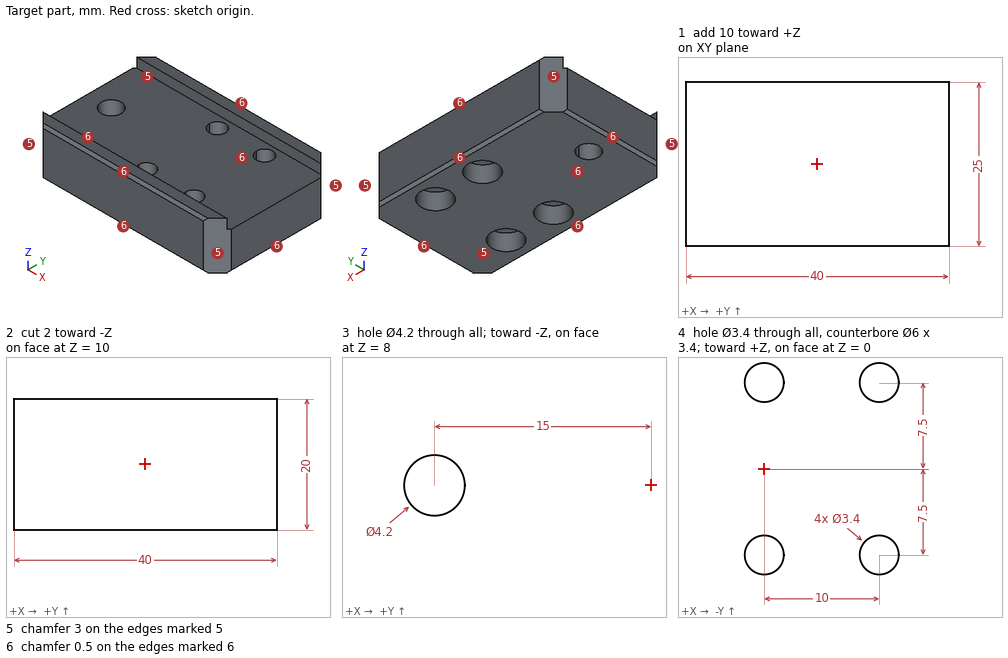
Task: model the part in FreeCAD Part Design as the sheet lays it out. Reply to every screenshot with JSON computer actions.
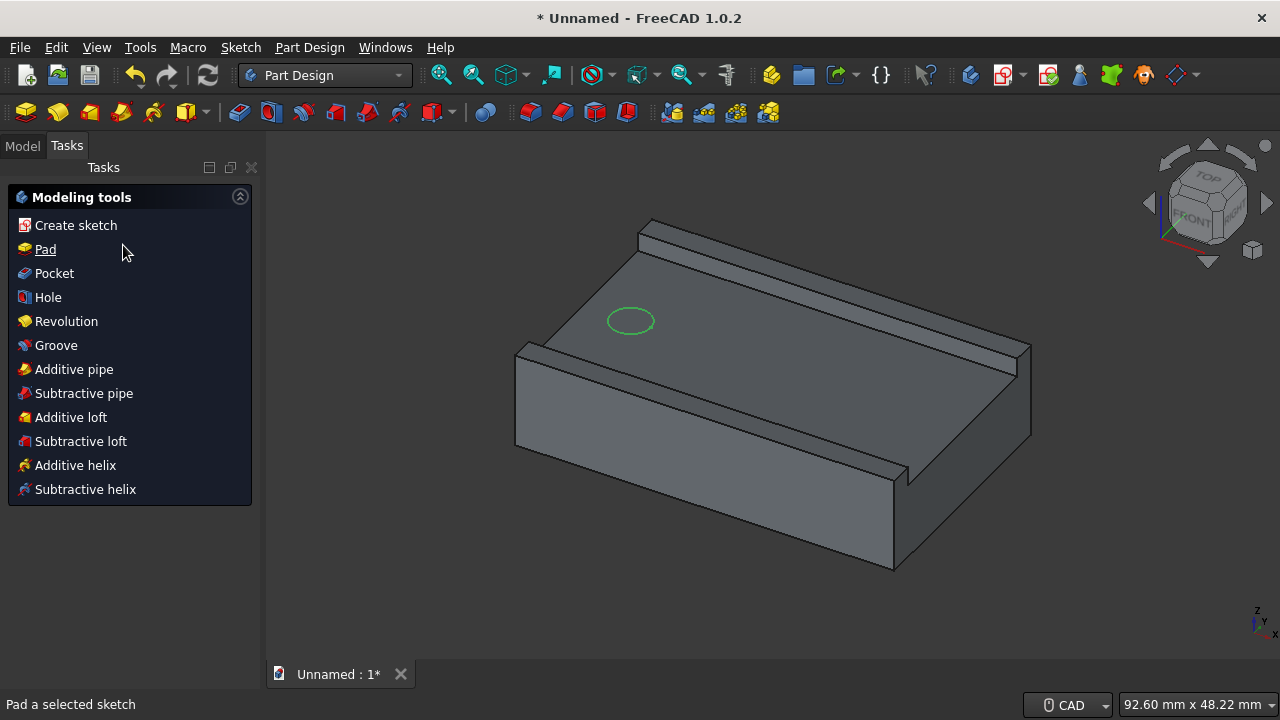
{"action": "left_click", "coordinate": [272, 112]}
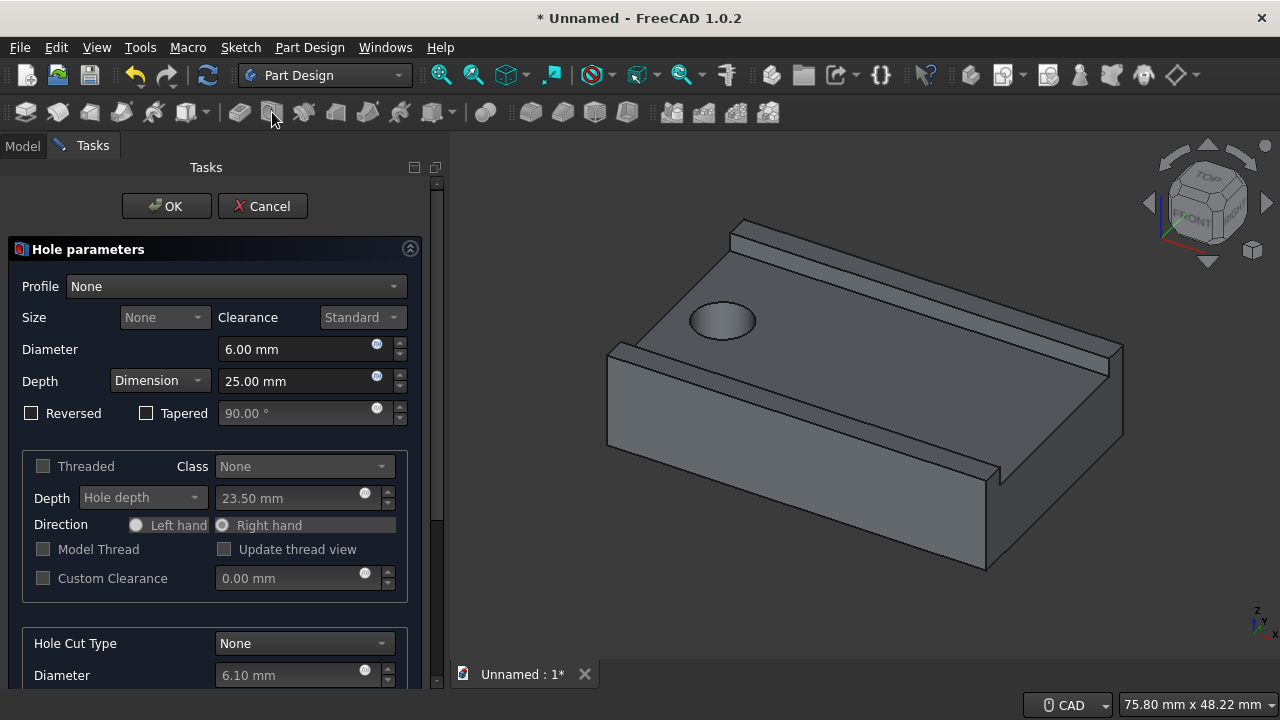
{"action": "triple_click", "coordinate": [305, 349]}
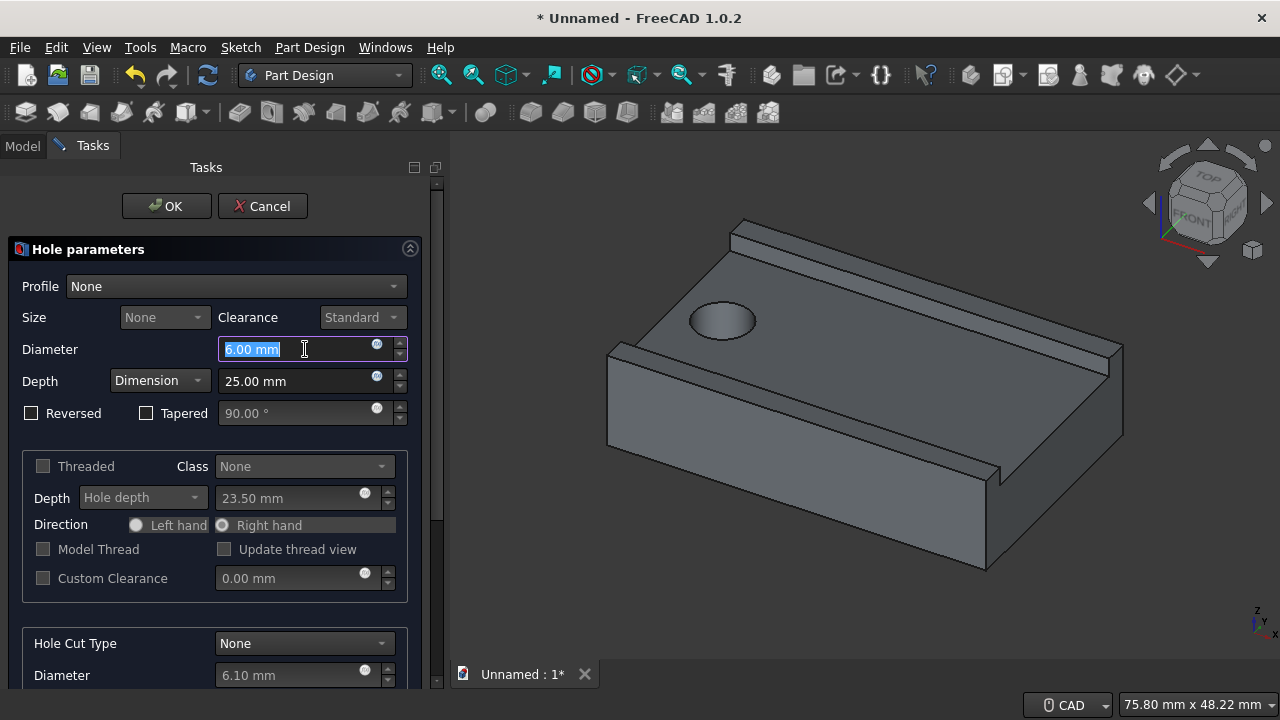
{"action": "type", "text": "4.2"}
{"action": "key", "text": "Tab"}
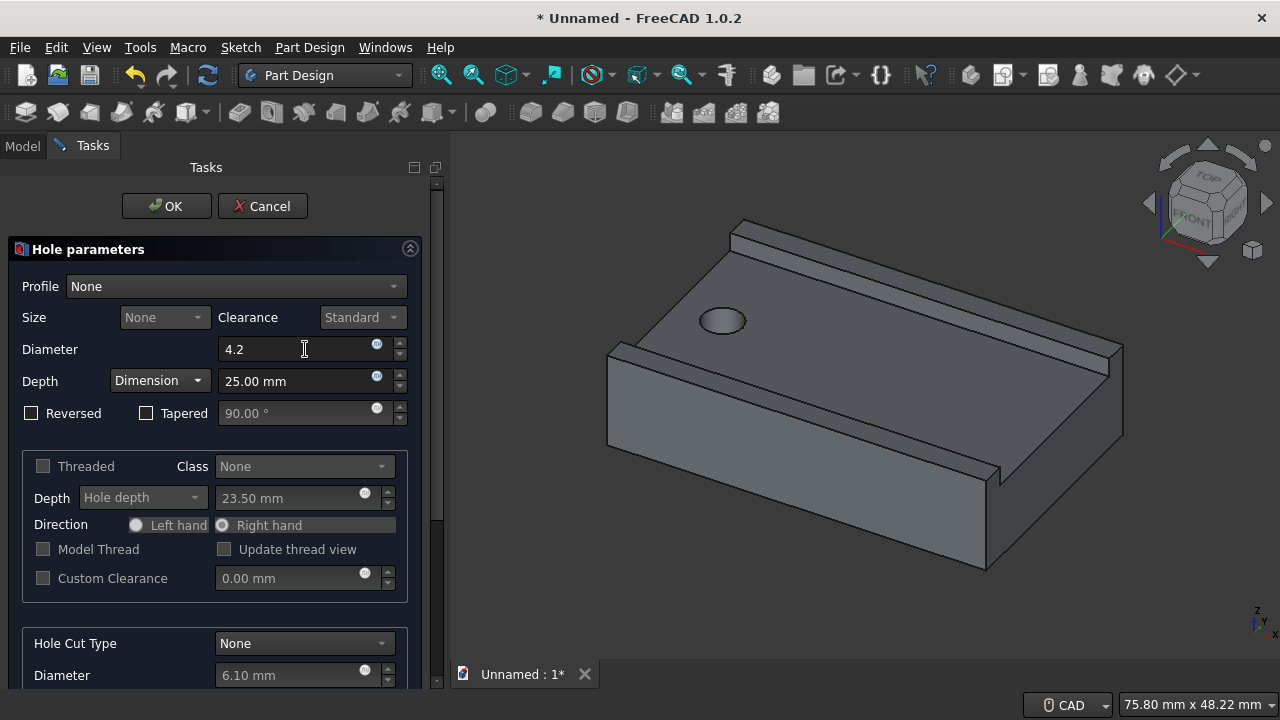
{"action": "left_click", "coordinate": [161, 380]}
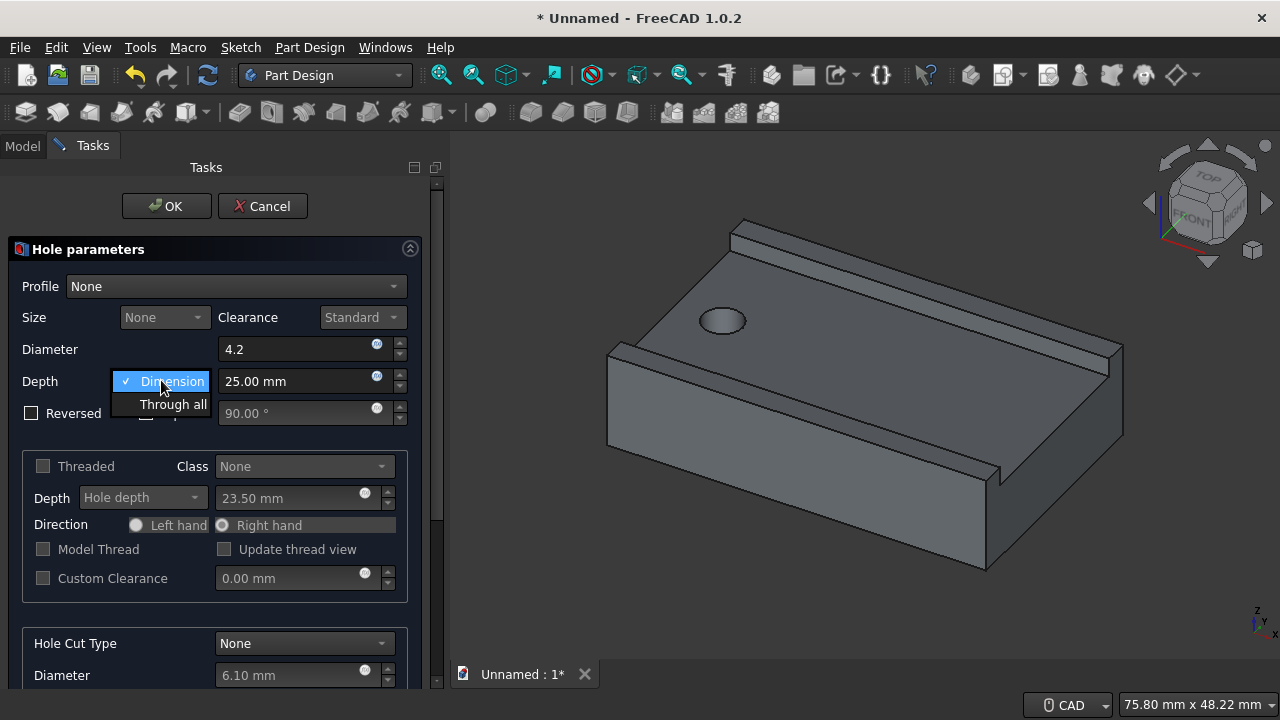
{"action": "left_click", "coordinate": [160, 404]}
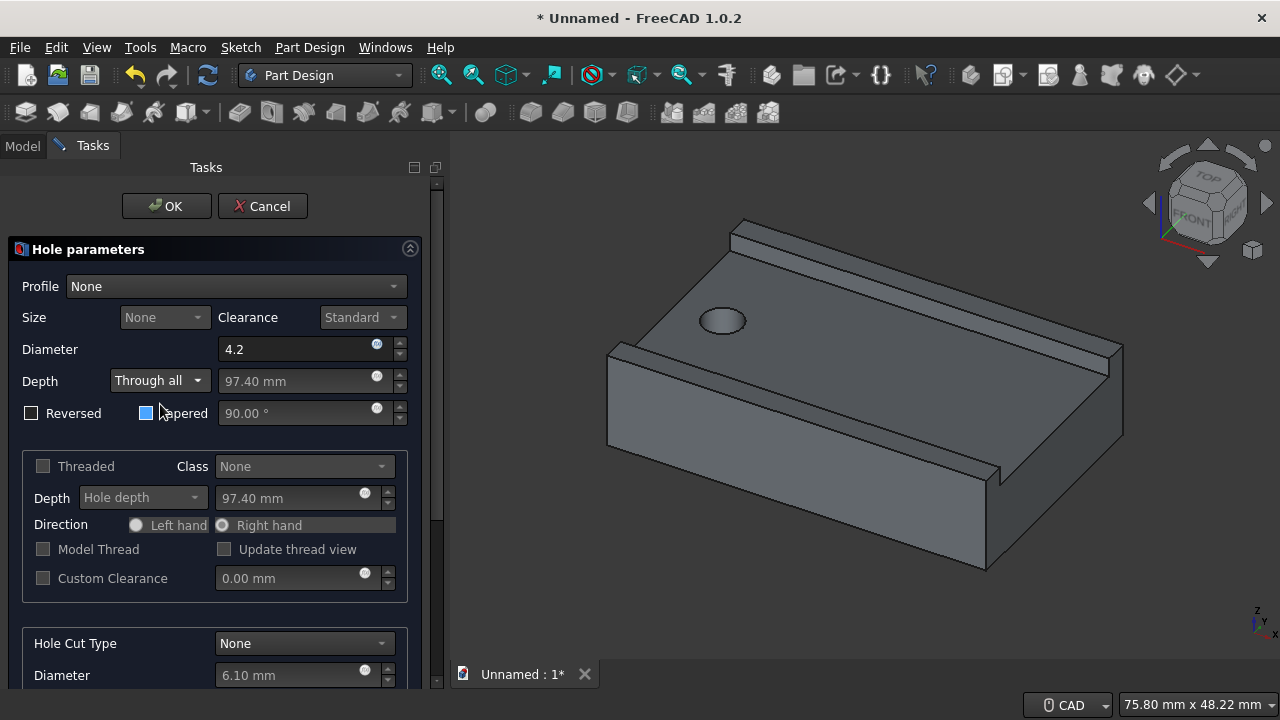
{"action": "left_click", "coordinate": [167, 206]}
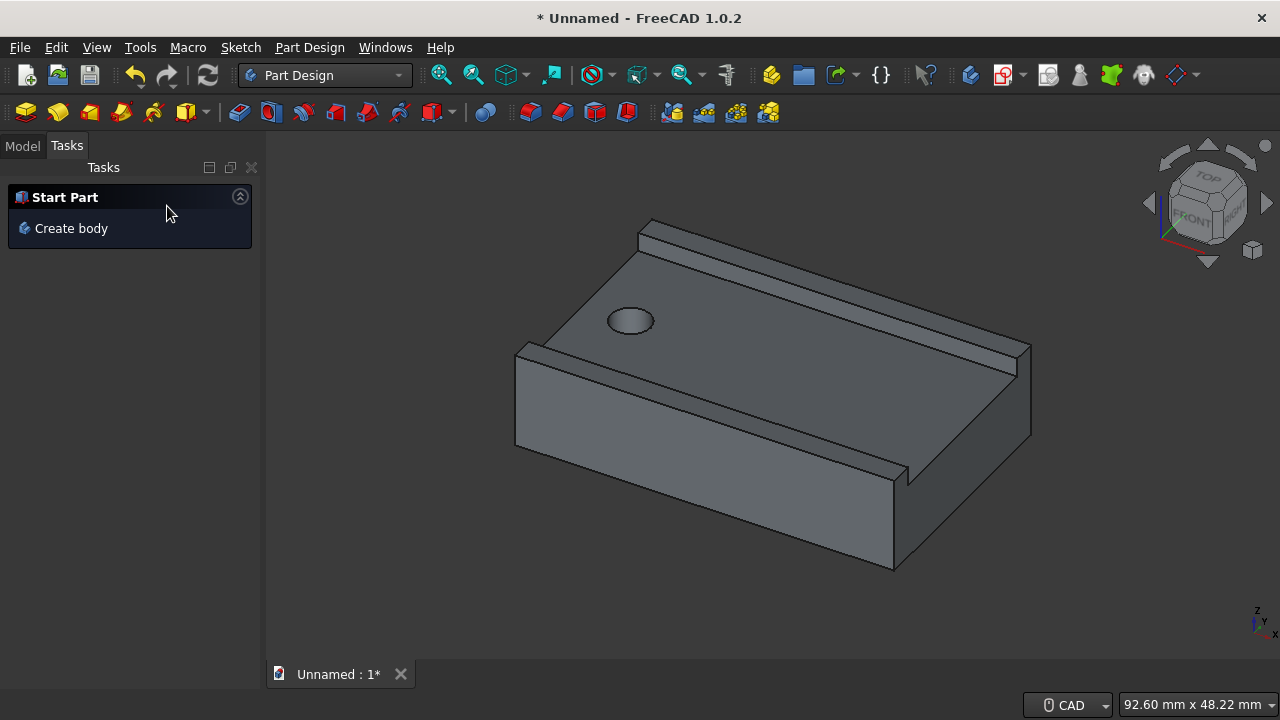
{"action": "key", "text": "5"}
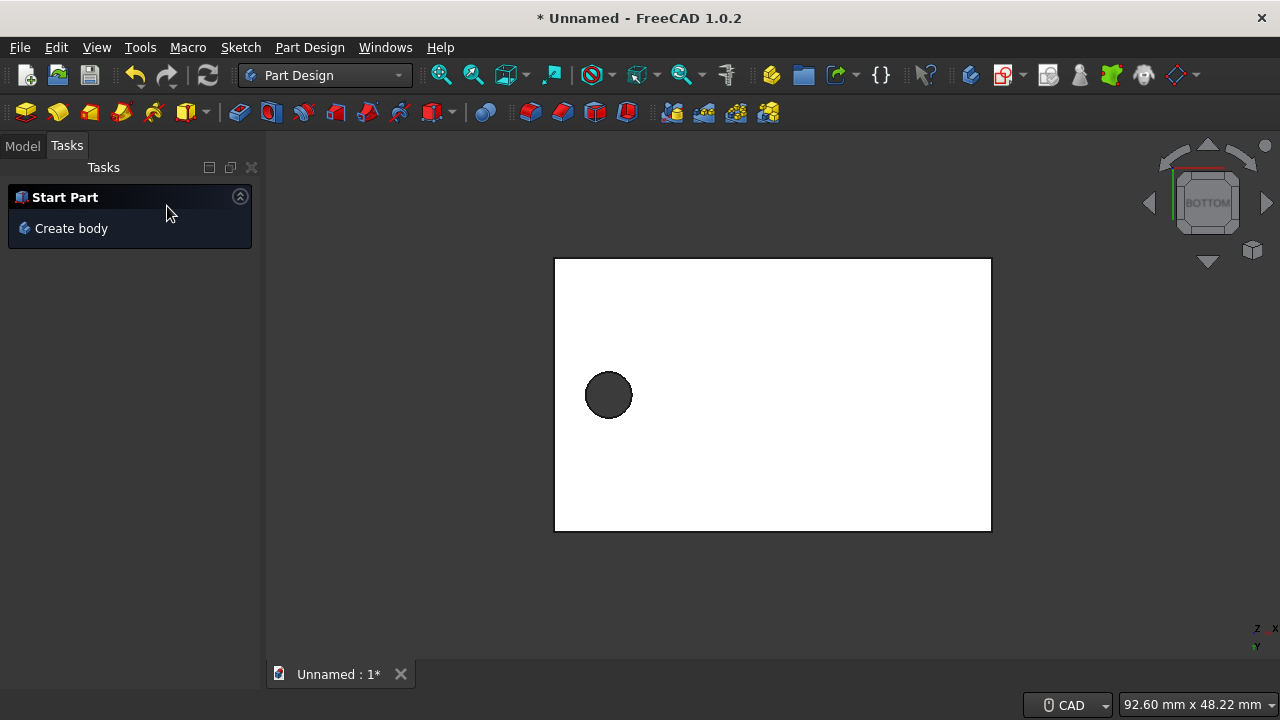
{"action": "left_click", "coordinate": [836, 394]}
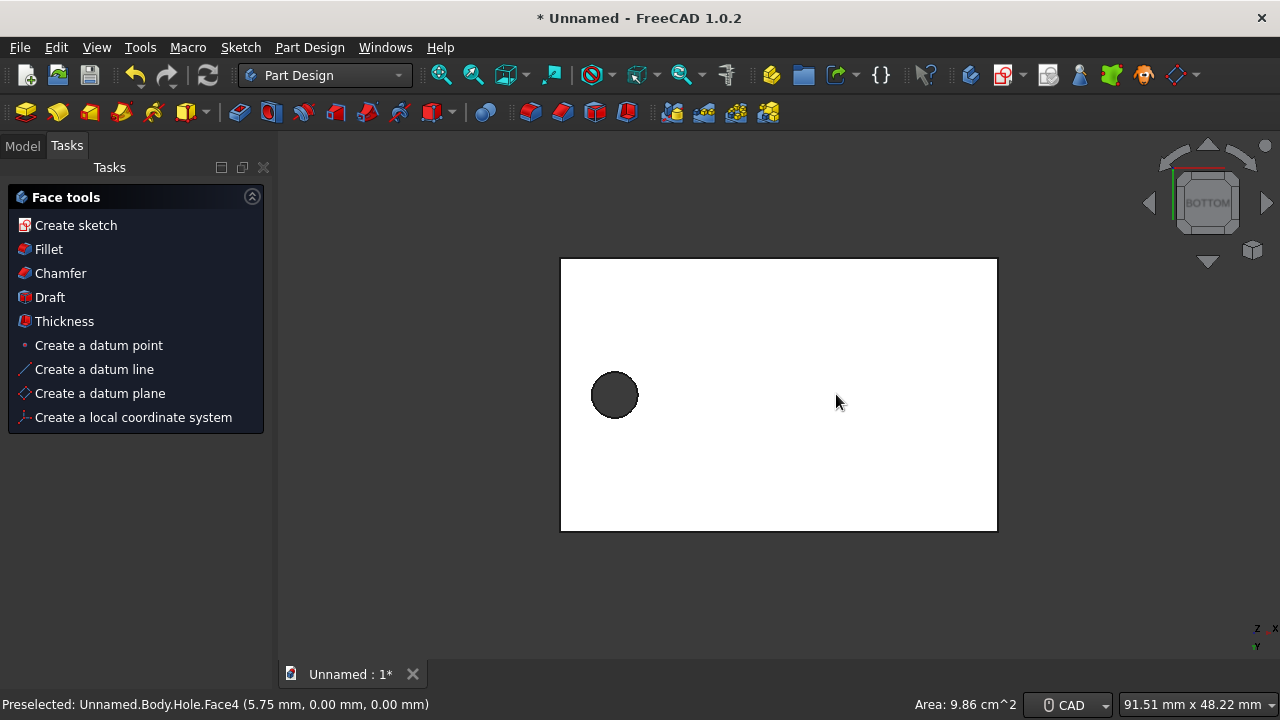
{"action": "left_click", "coordinate": [1004, 76]}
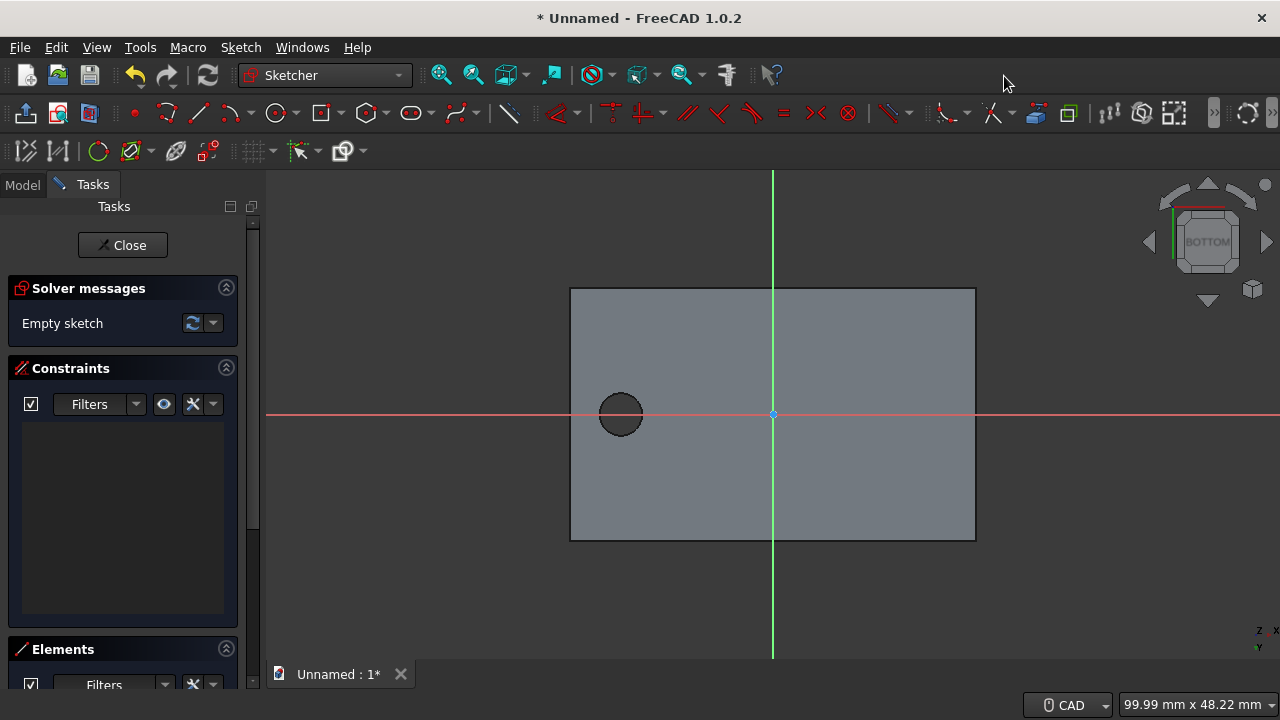
{"action": "scroll", "coordinate": [1066, 414], "scroll_direction": "up", "scroll_amount": 2}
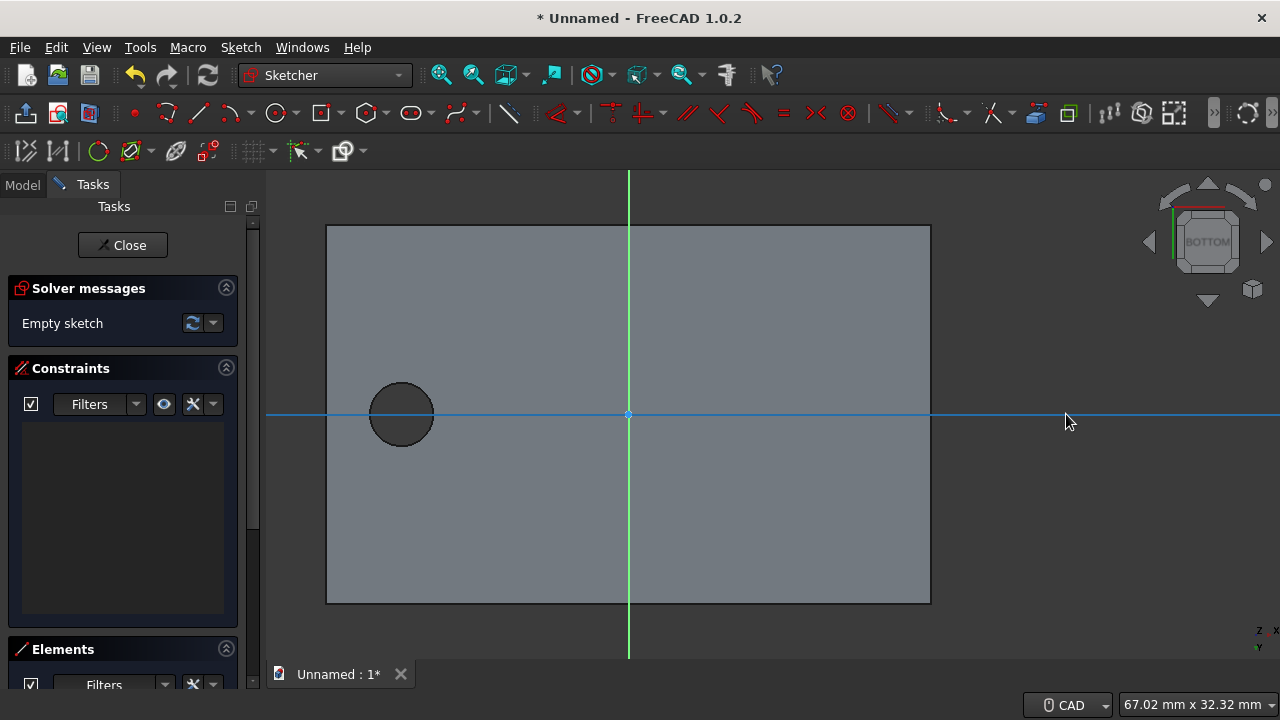
{"action": "left_click", "coordinate": [276, 114]}